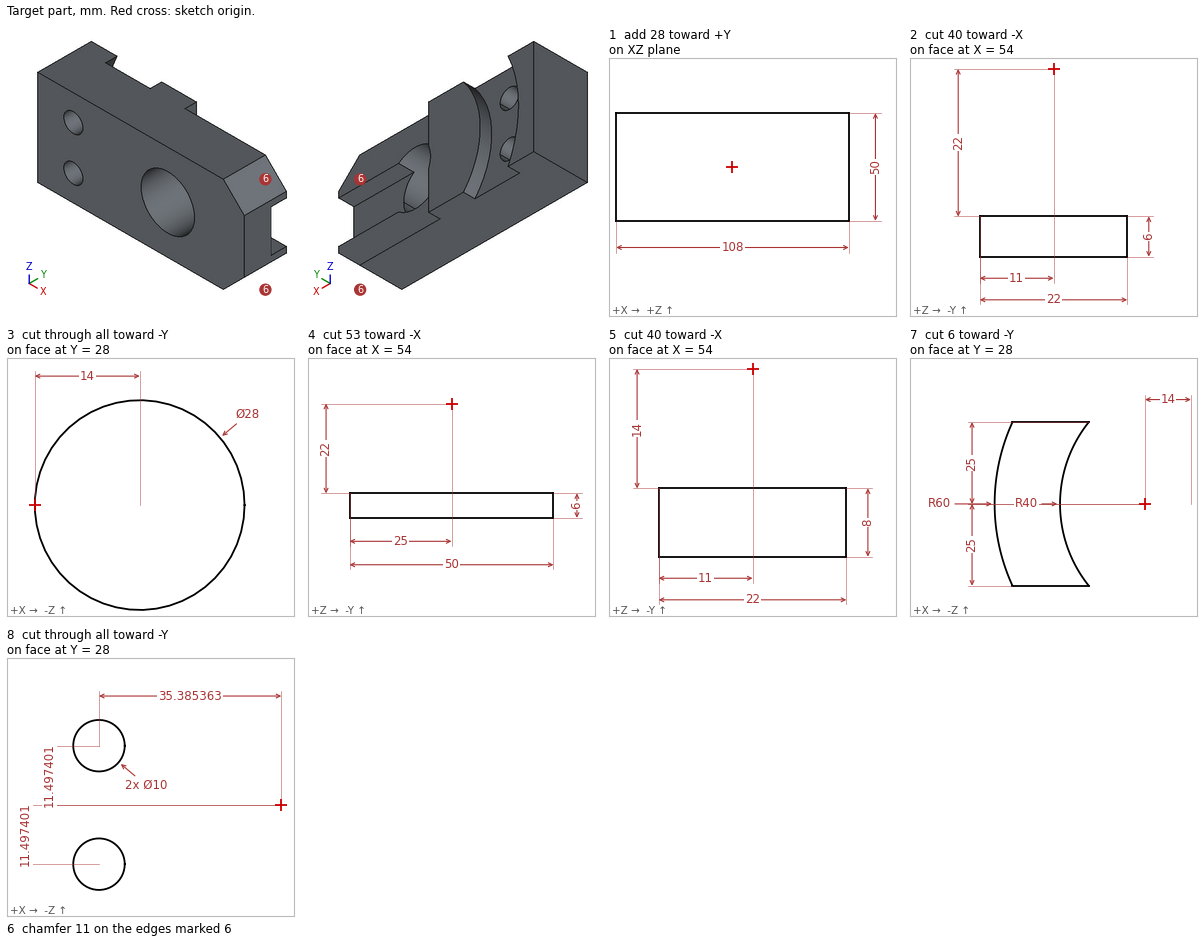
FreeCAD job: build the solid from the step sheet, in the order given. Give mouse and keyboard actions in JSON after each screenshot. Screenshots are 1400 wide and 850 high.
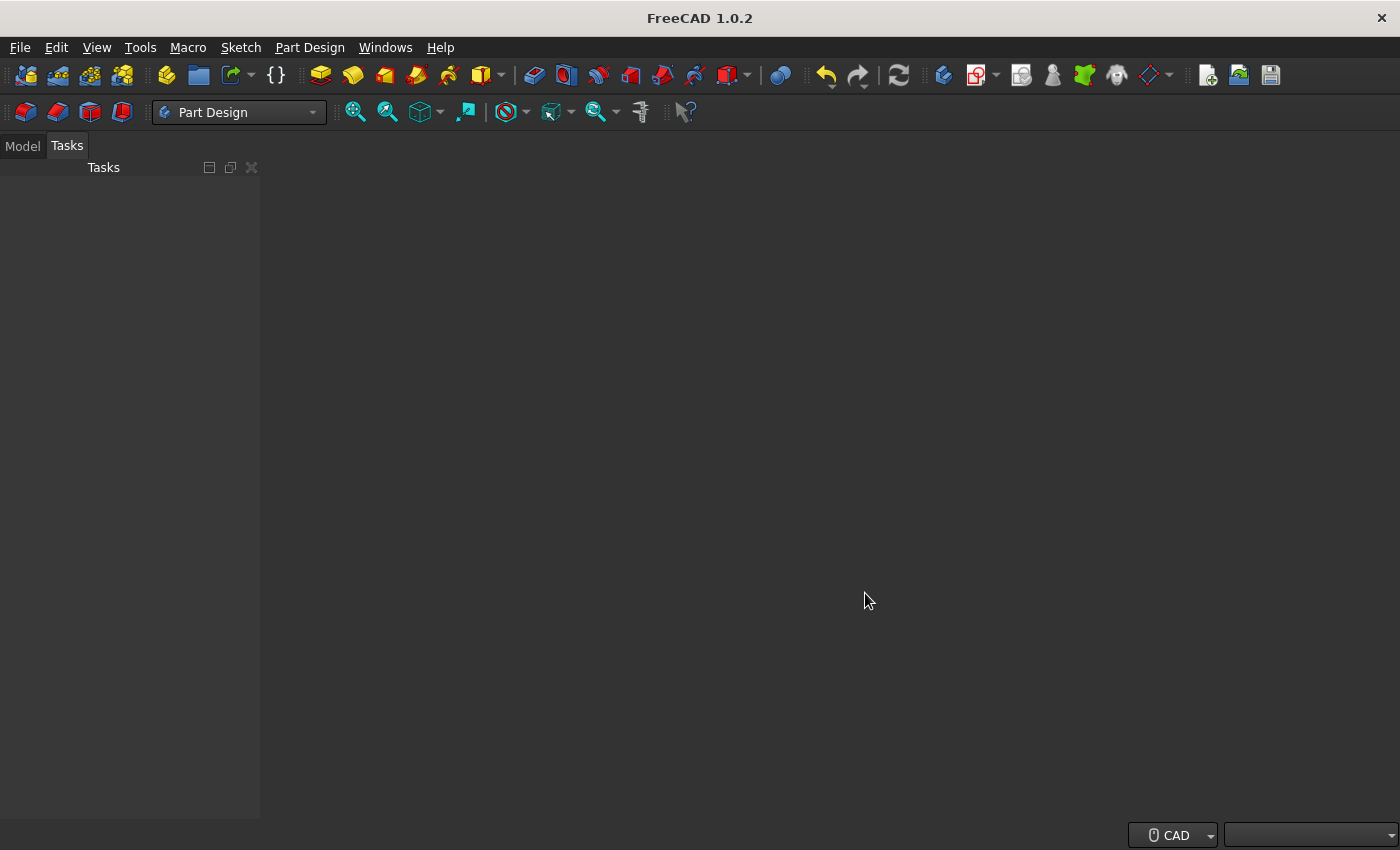
{"action": "left_click", "coordinate": [1208, 76]}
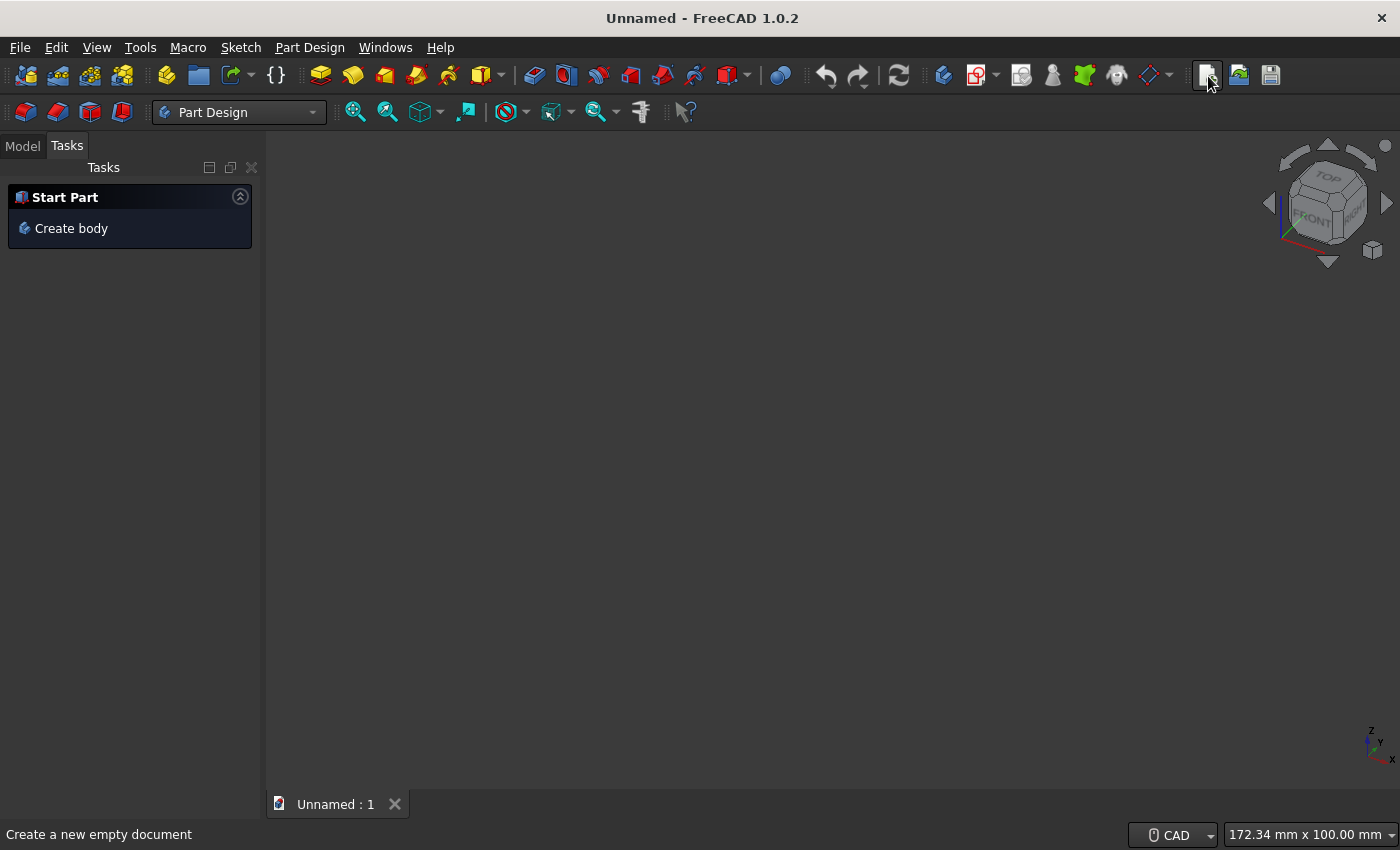
{"action": "left_click", "coordinate": [976, 76]}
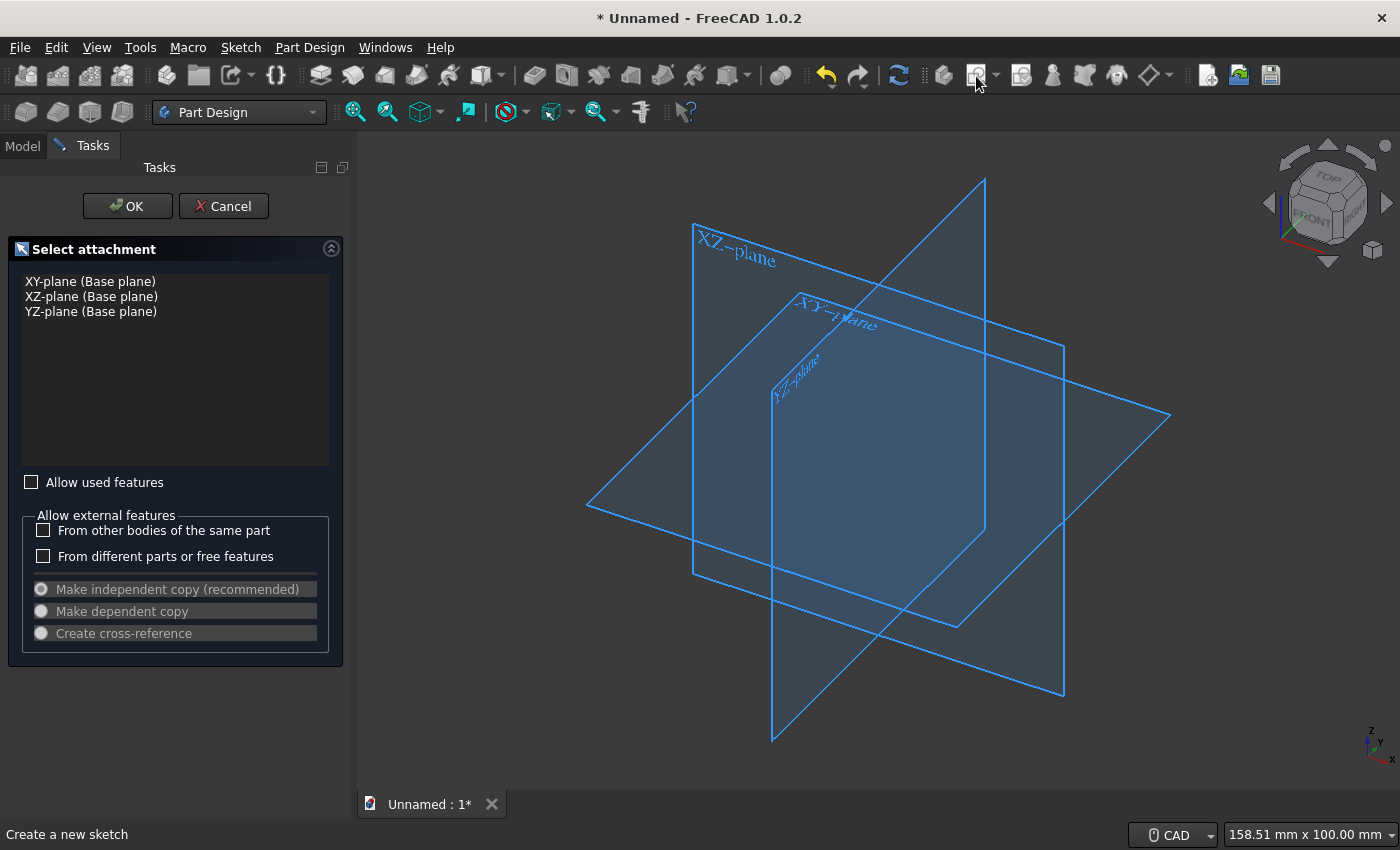
{"action": "left_click", "coordinate": [82, 296]}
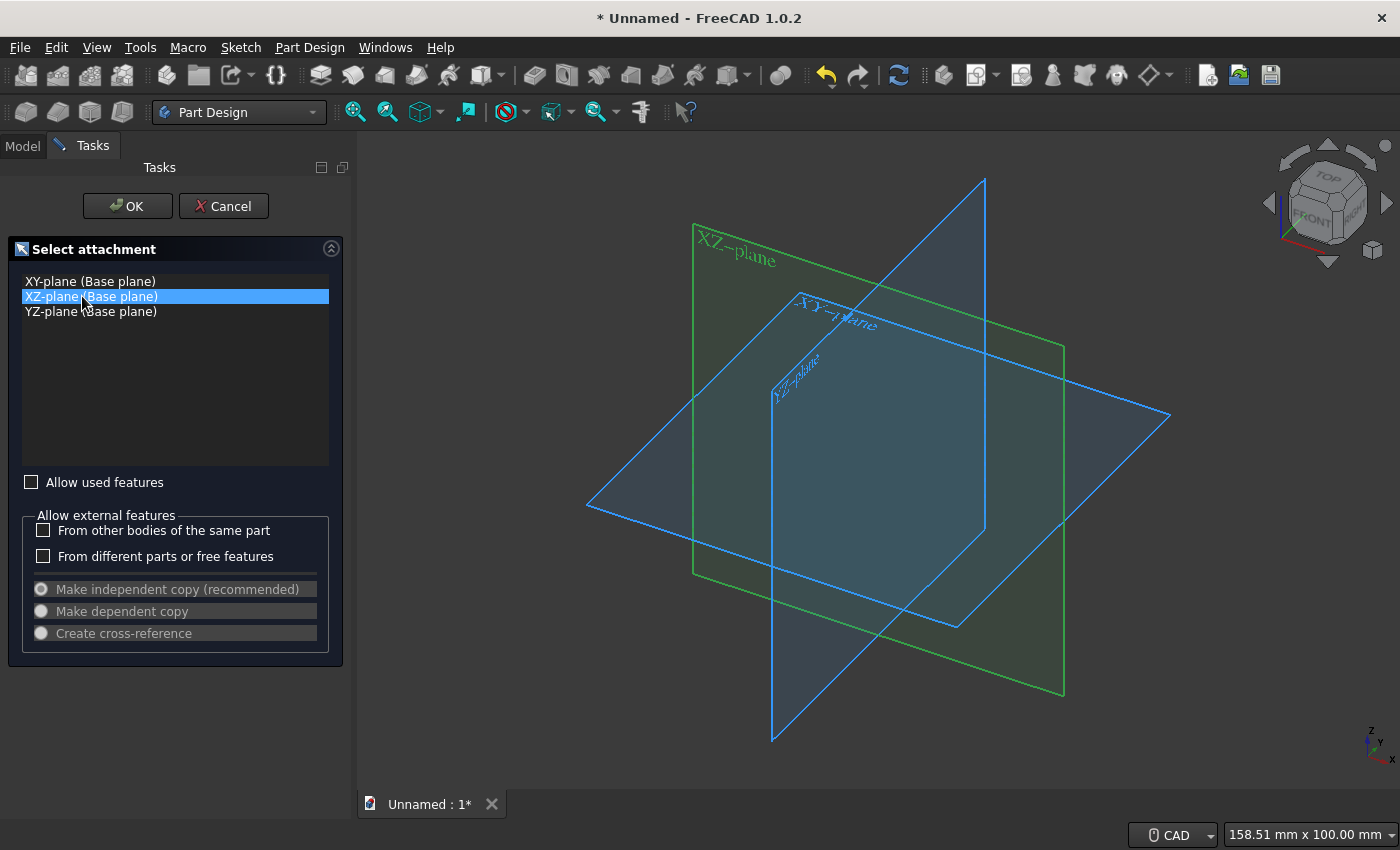
{"action": "left_click", "coordinate": [128, 206]}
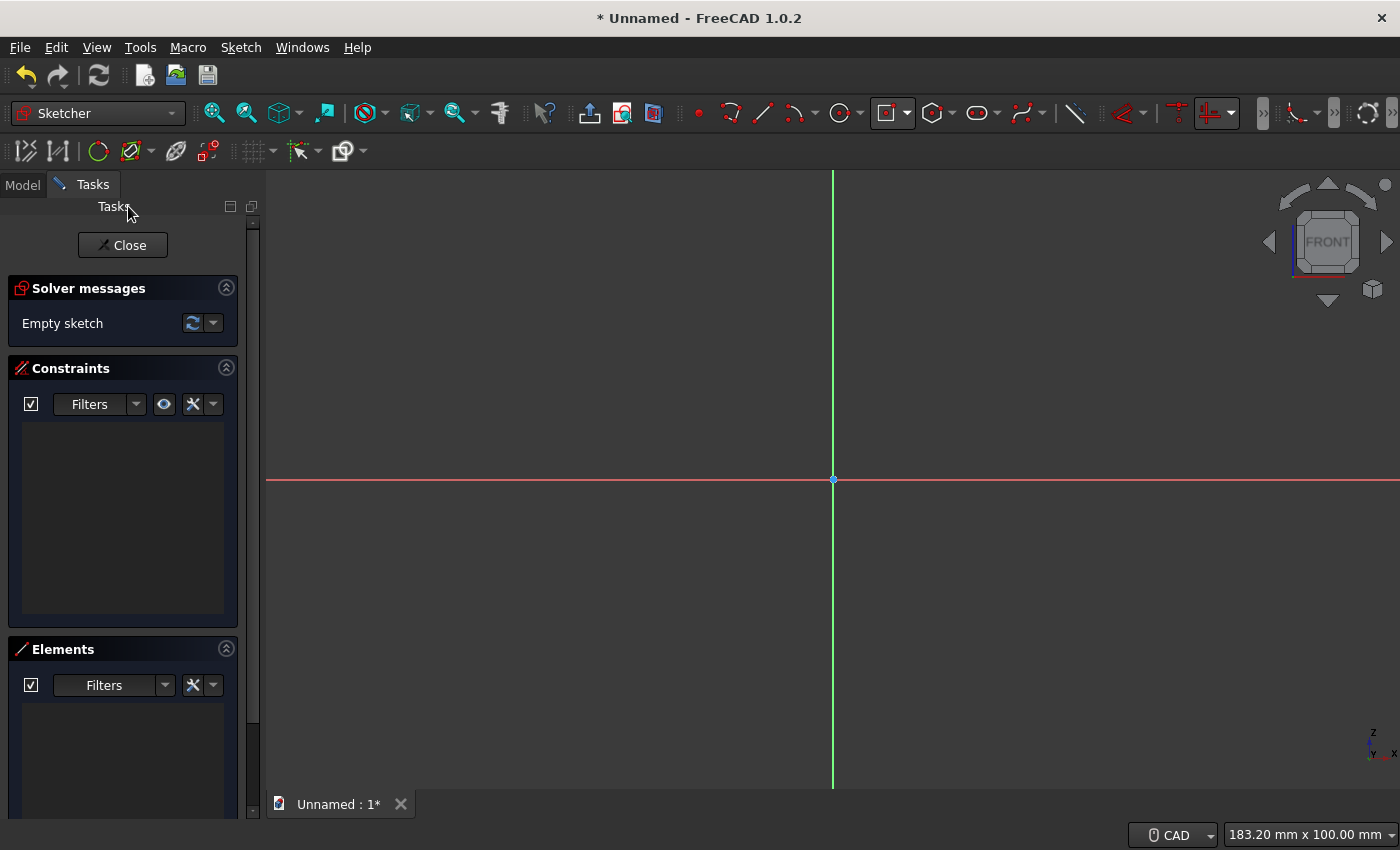
{"action": "left_click", "coordinate": [886, 114]}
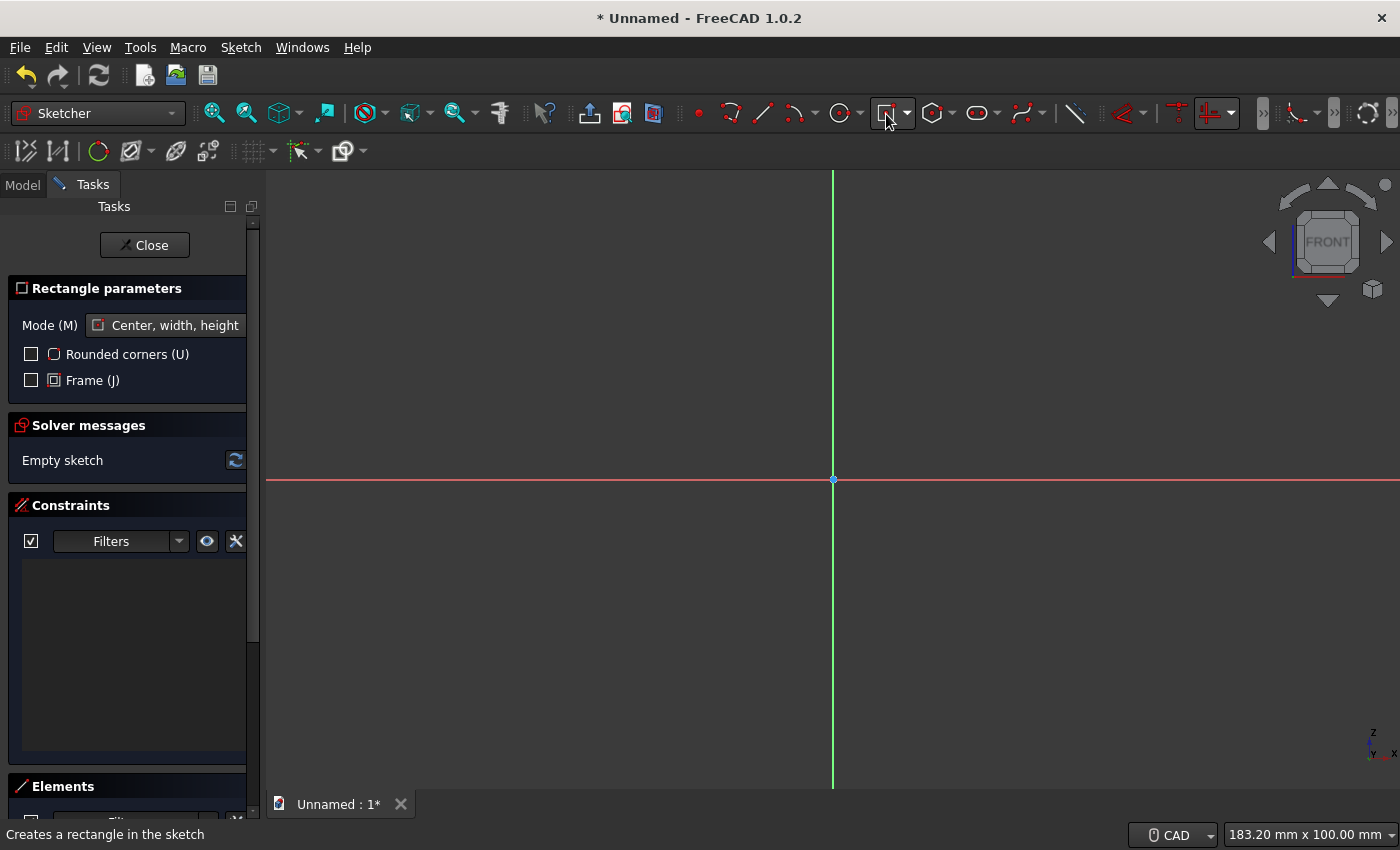
{"action": "left_click", "coordinate": [833, 480]}
{"action": "mouse_move", "coordinate": [1167, 325]}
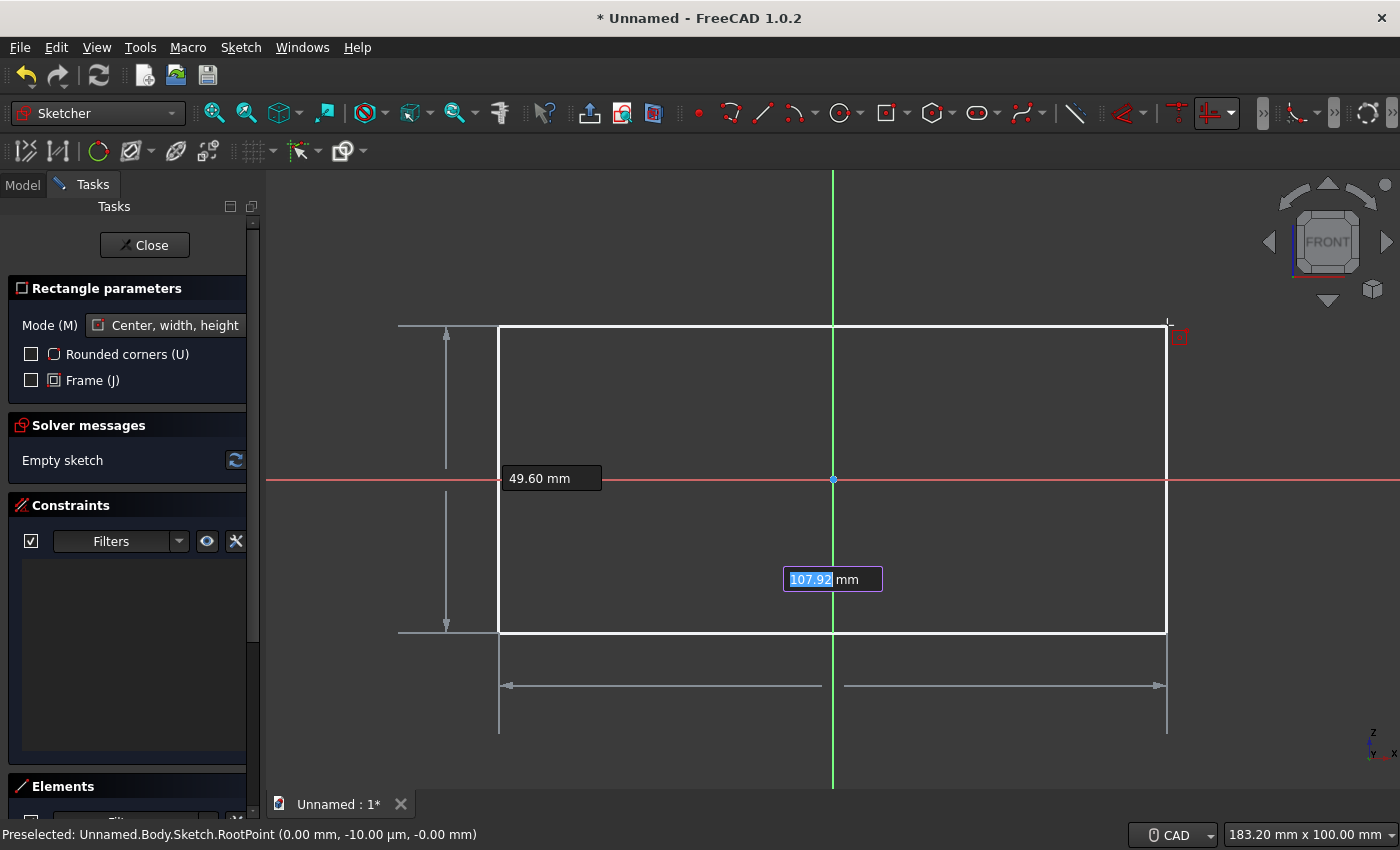
{"action": "type", "text": "108"}
{"action": "key", "text": "Tab"}
{"action": "type", "text": "50"}
{"action": "key", "text": "Return"}
{"action": "key", "text": "Escape"}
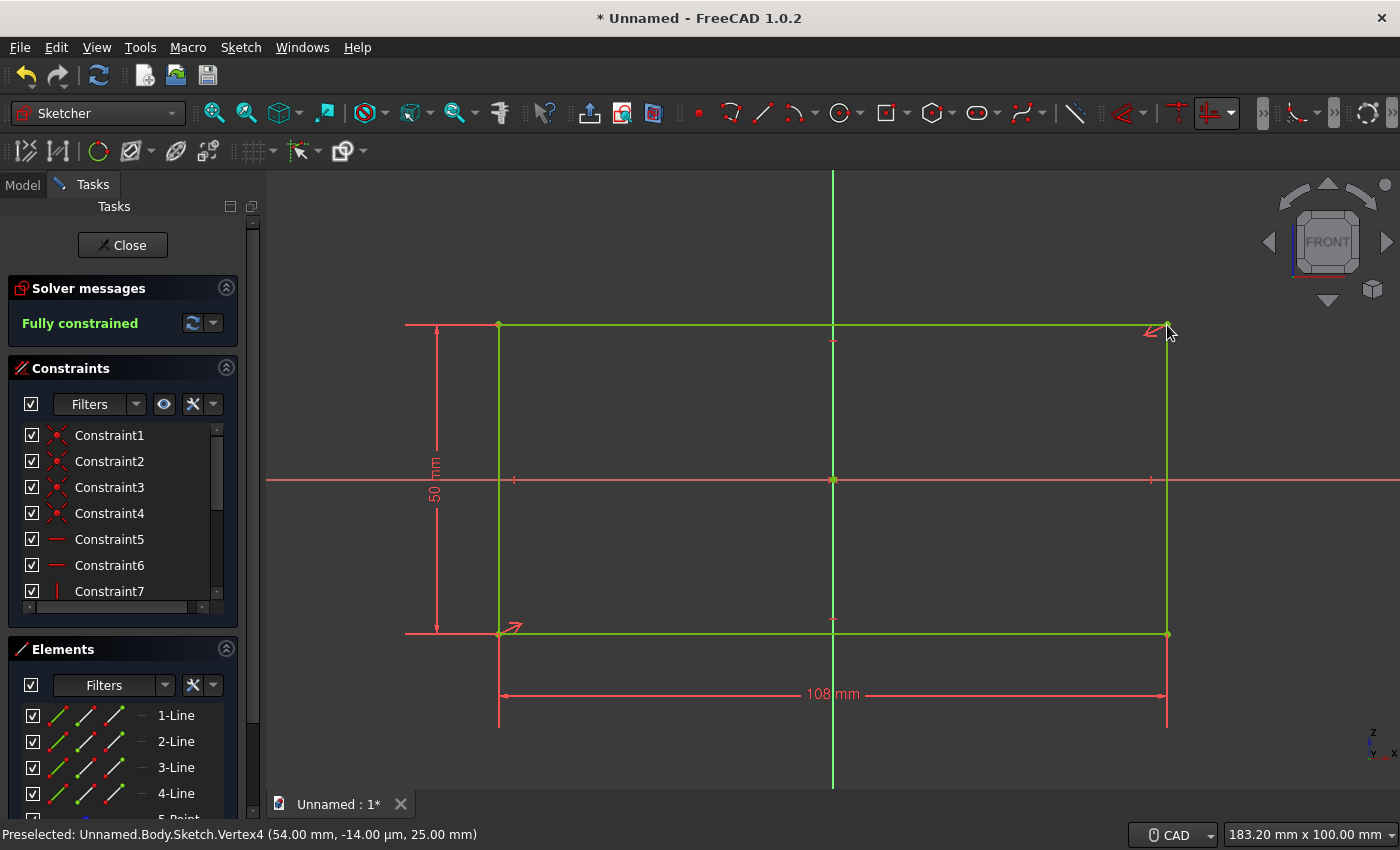
{"action": "left_click", "coordinate": [123, 245]}